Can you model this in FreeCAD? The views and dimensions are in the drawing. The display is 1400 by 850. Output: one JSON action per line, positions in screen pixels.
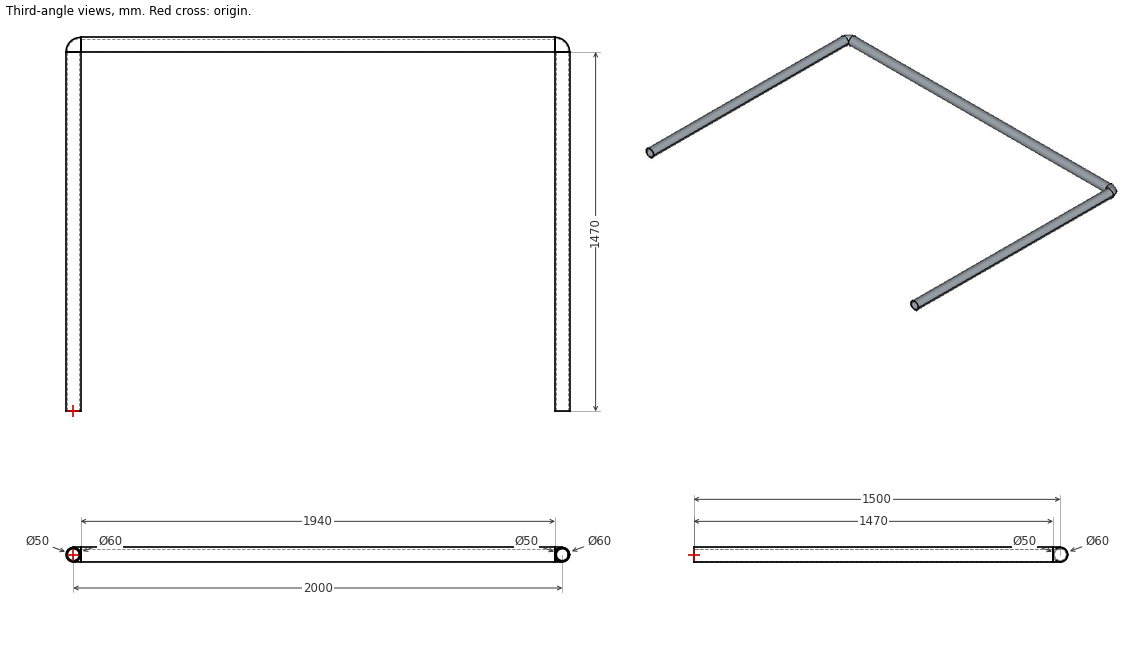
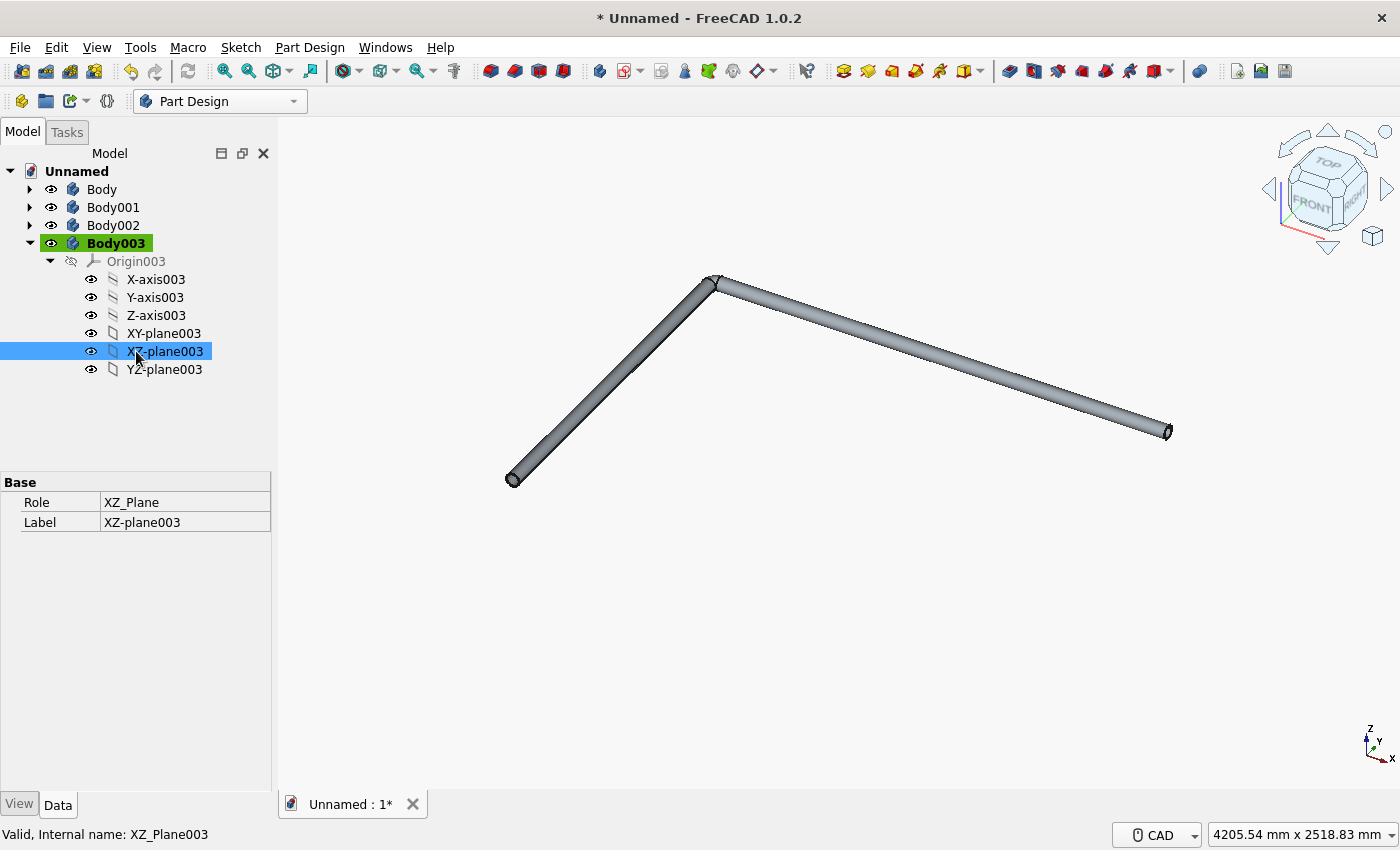
{"action": "left_click", "coordinate": [758, 72]}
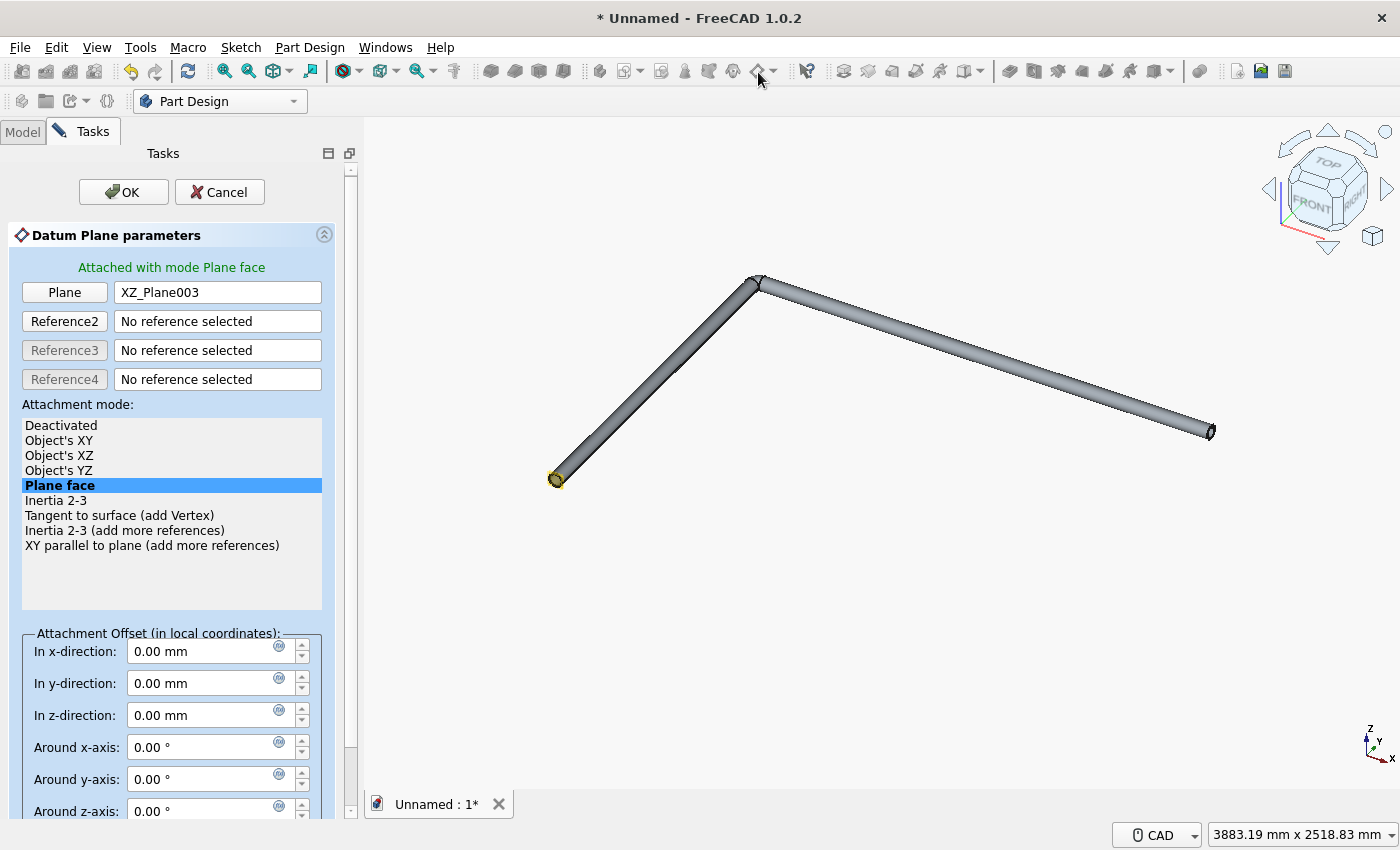
{"action": "triple_click", "coordinate": [210, 715]}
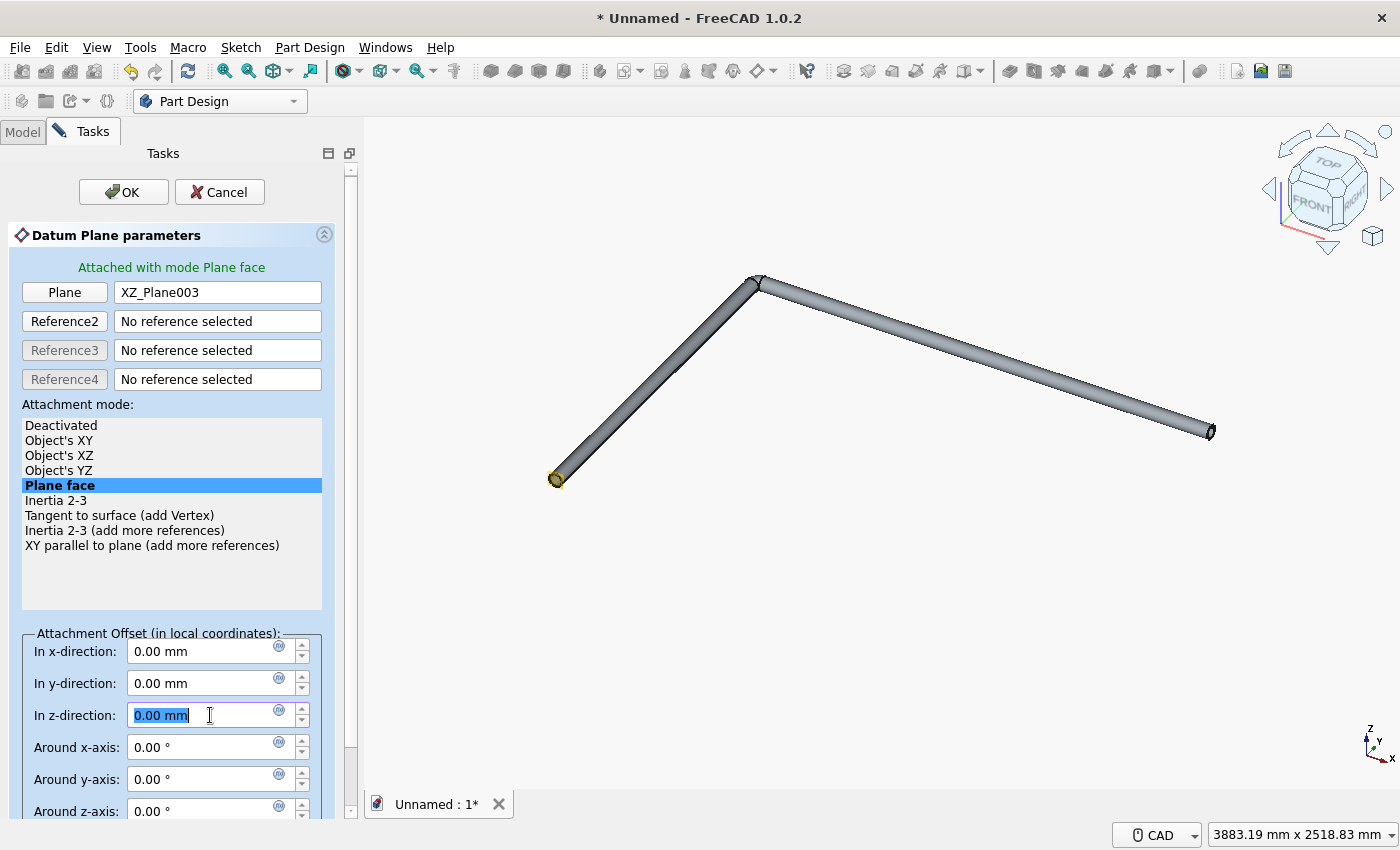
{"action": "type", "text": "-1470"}
{"action": "key", "text": "Tab"}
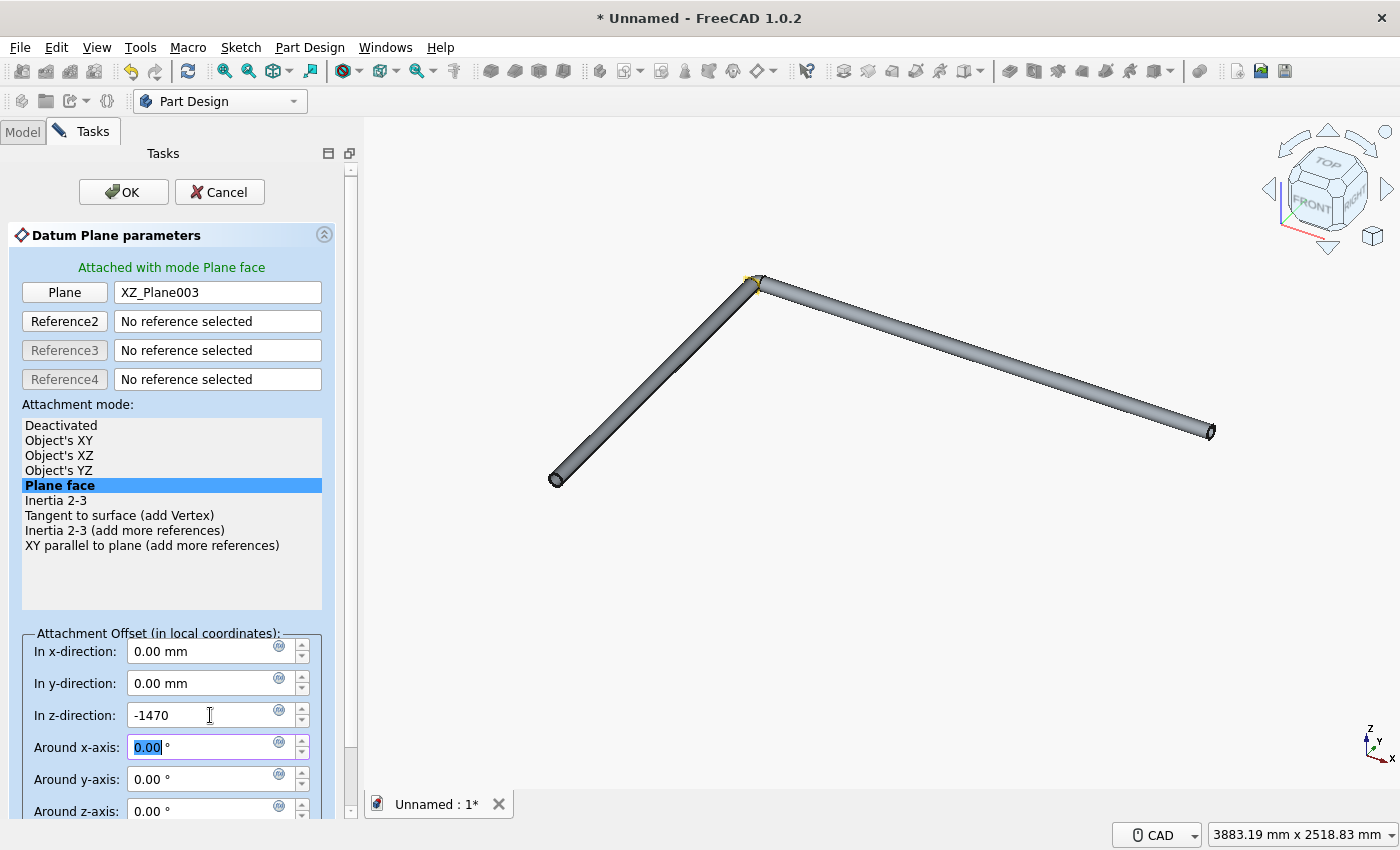
{"action": "left_click", "coordinate": [124, 192]}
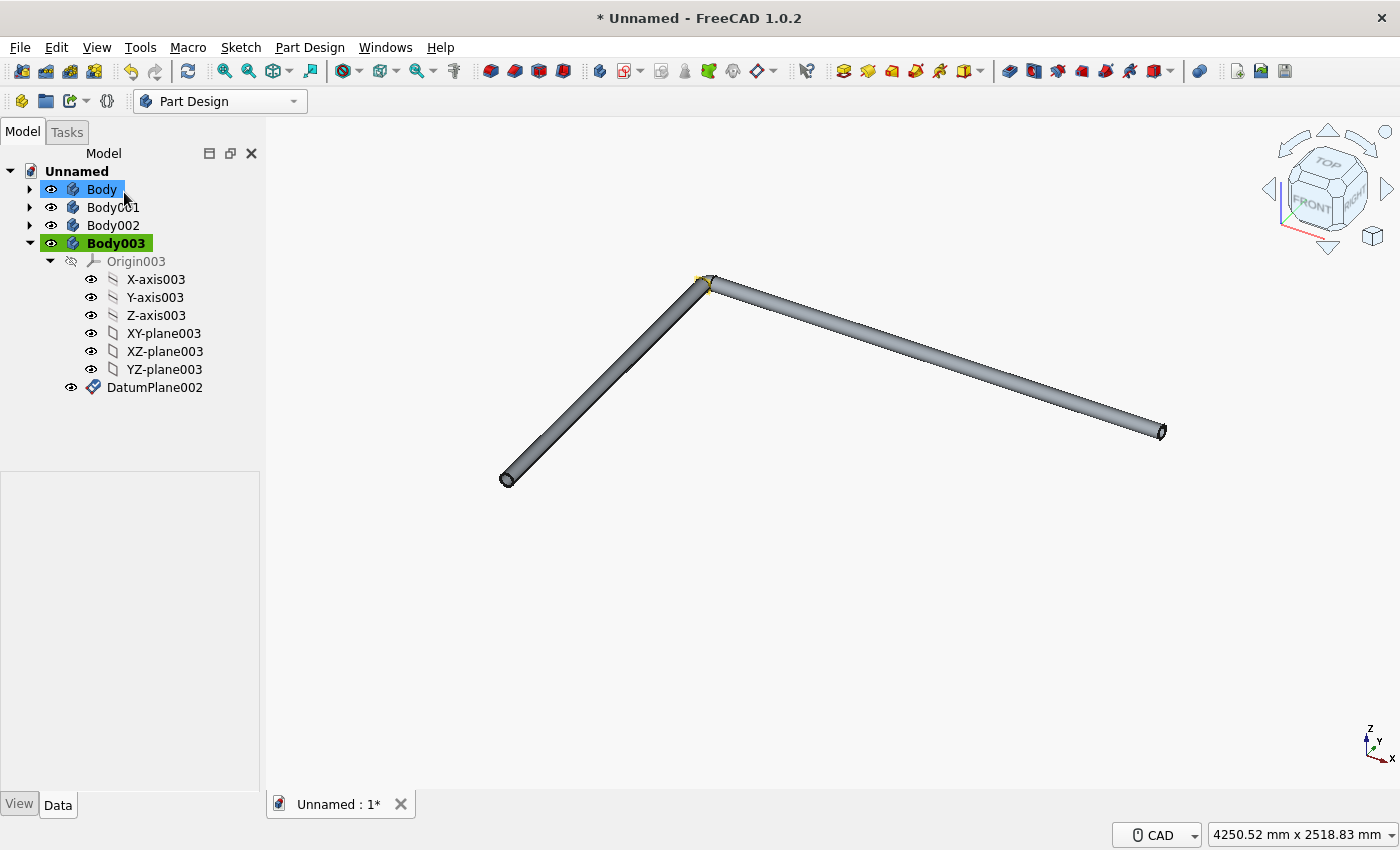
{"action": "left_click", "coordinate": [116, 387]}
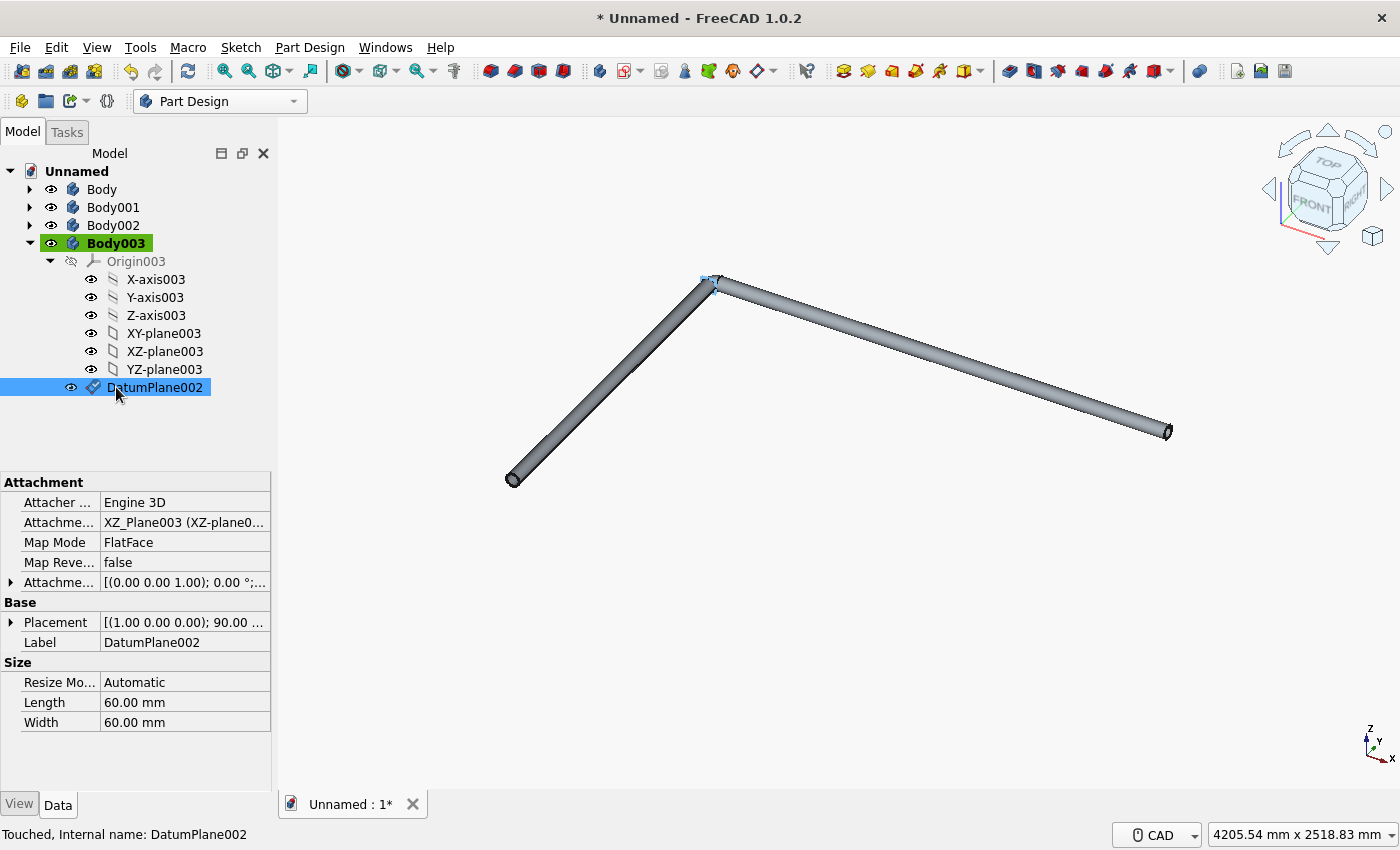
{"action": "left_click", "coordinate": [624, 72]}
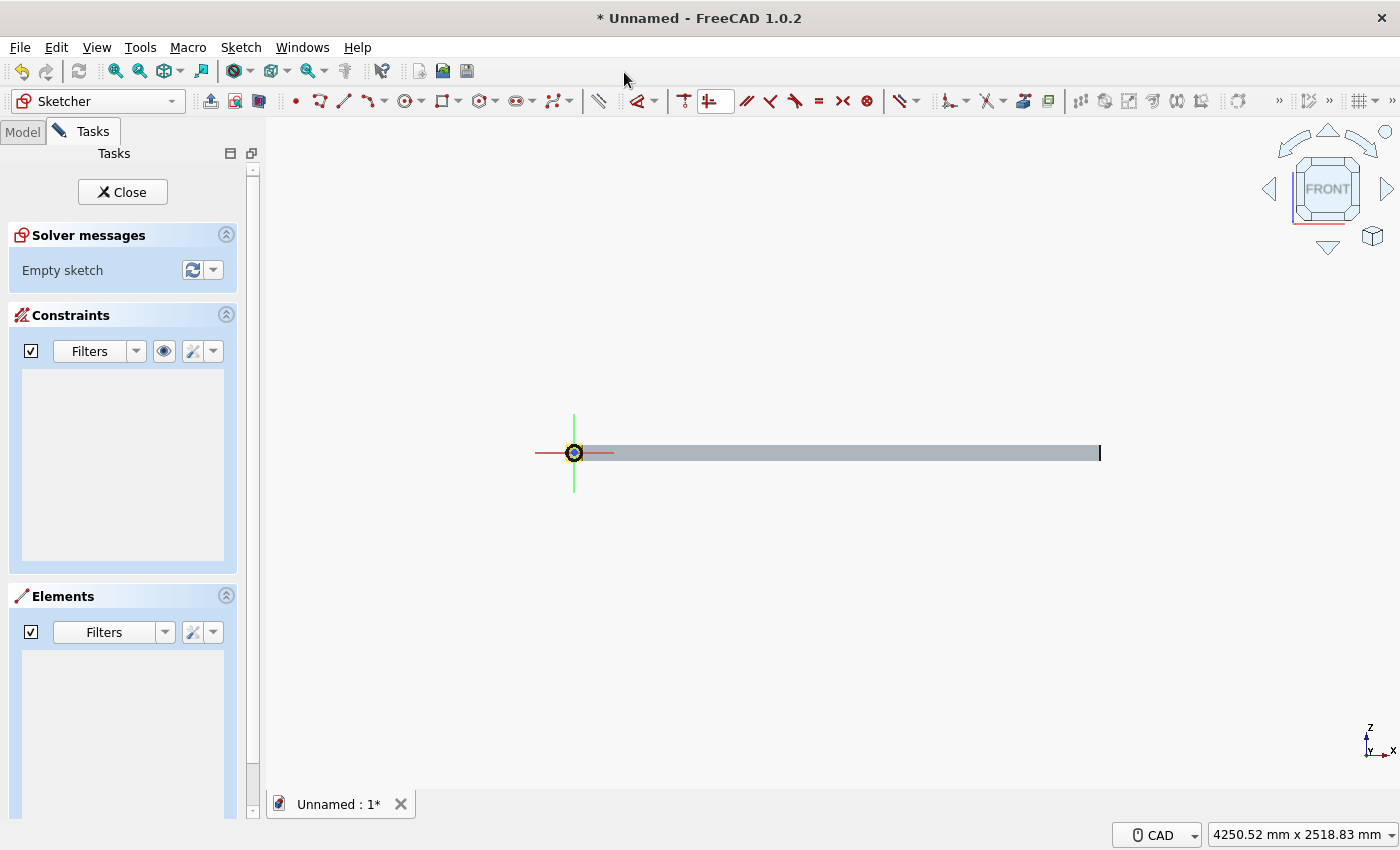
{"action": "scroll", "coordinate": [1126, 453], "scroll_direction": "up", "scroll_amount": 15}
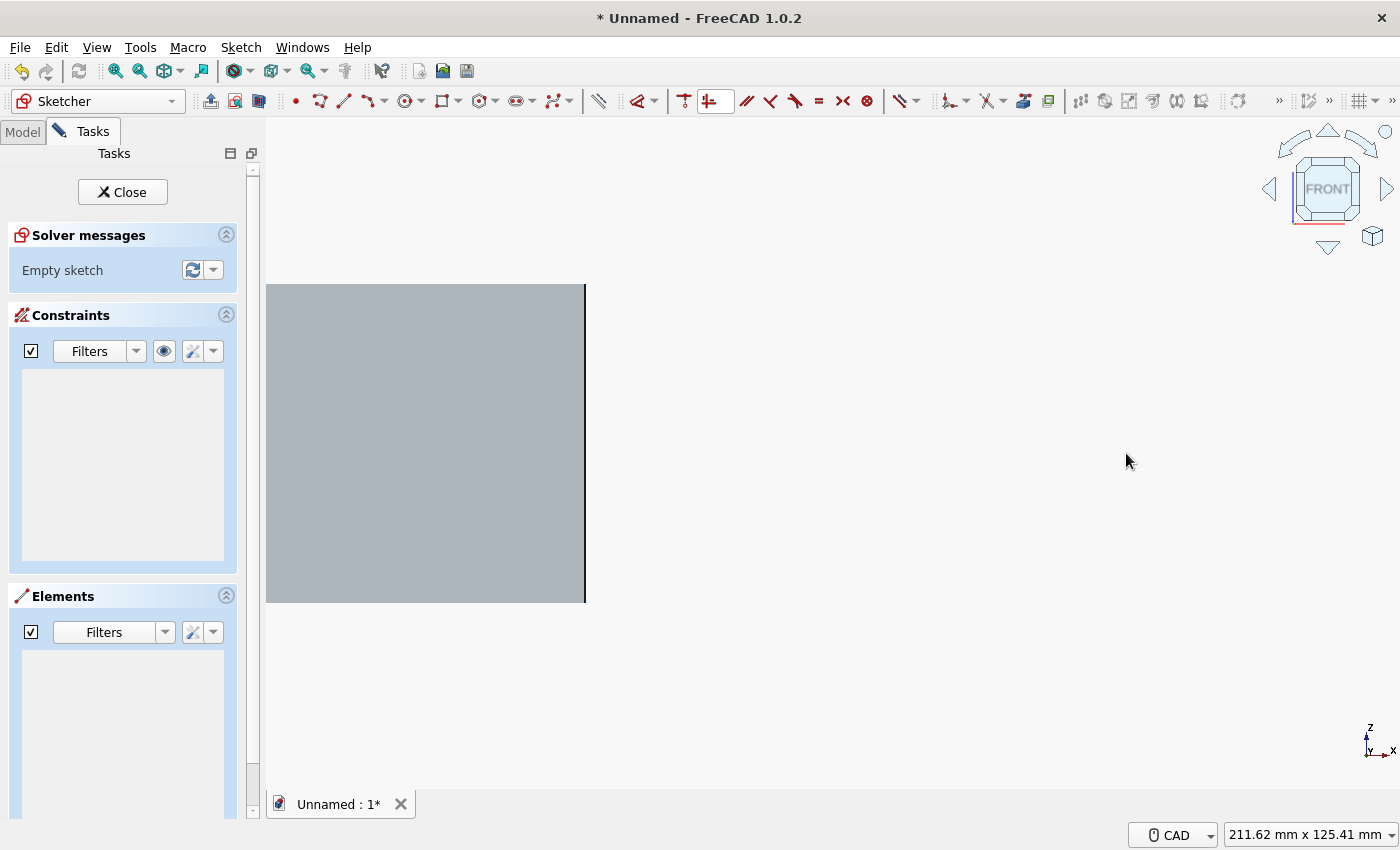
{"action": "key", "text": "g c"}